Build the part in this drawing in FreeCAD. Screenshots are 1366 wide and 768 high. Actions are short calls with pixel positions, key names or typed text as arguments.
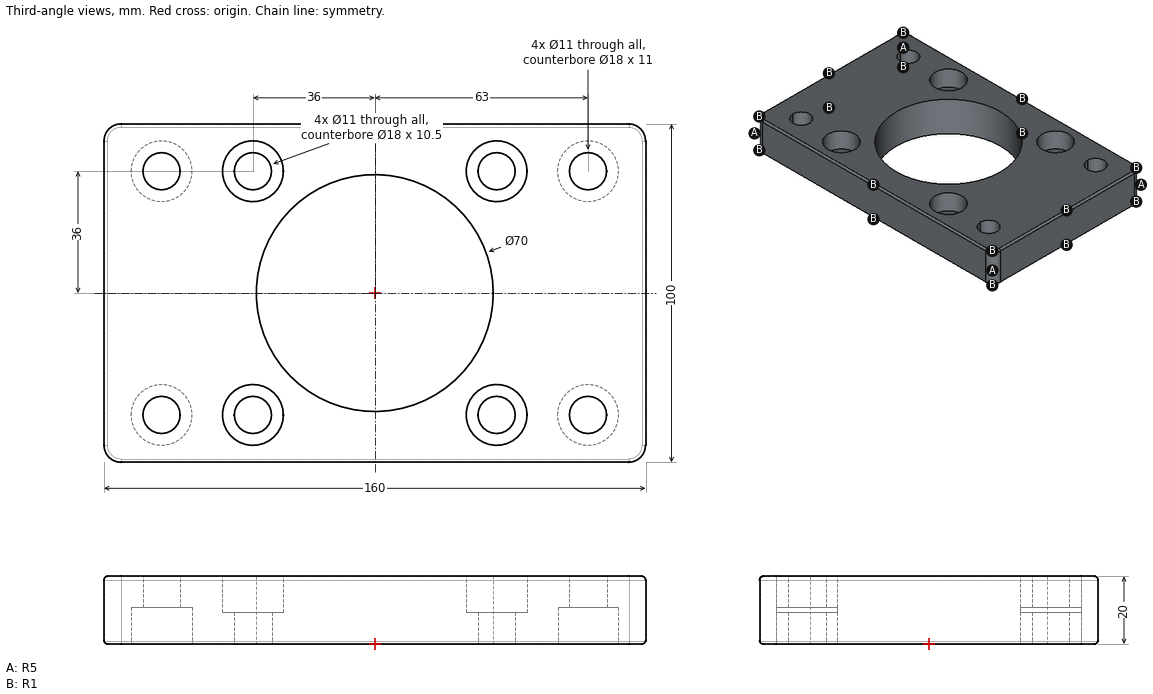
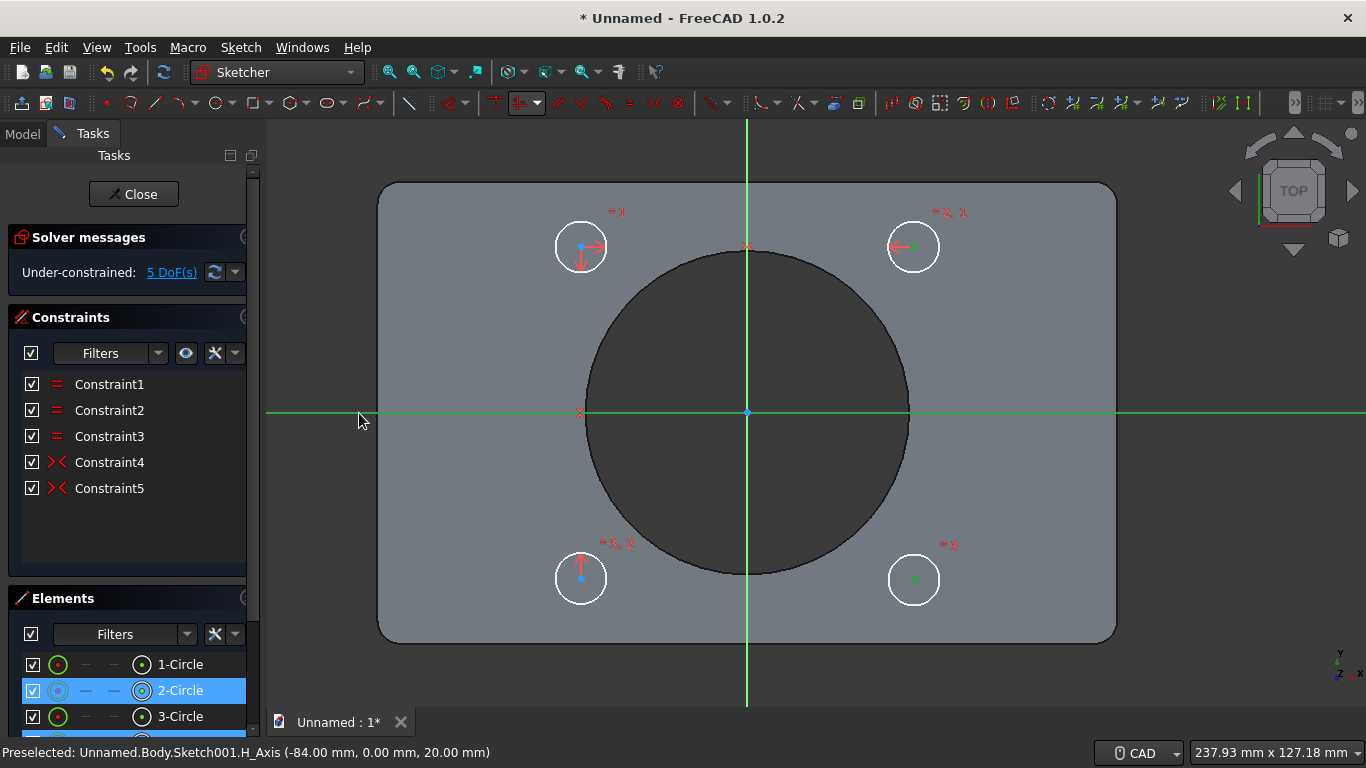
key(s)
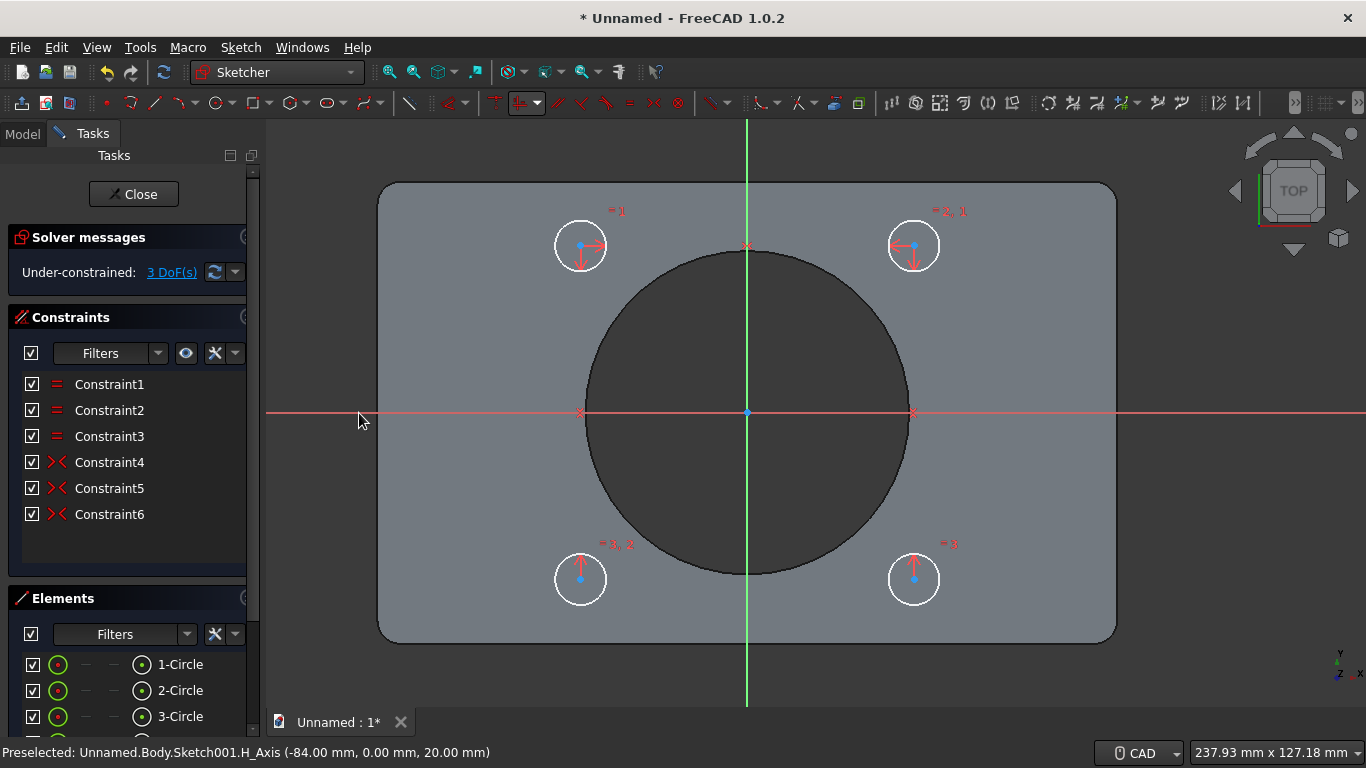
click(448, 104)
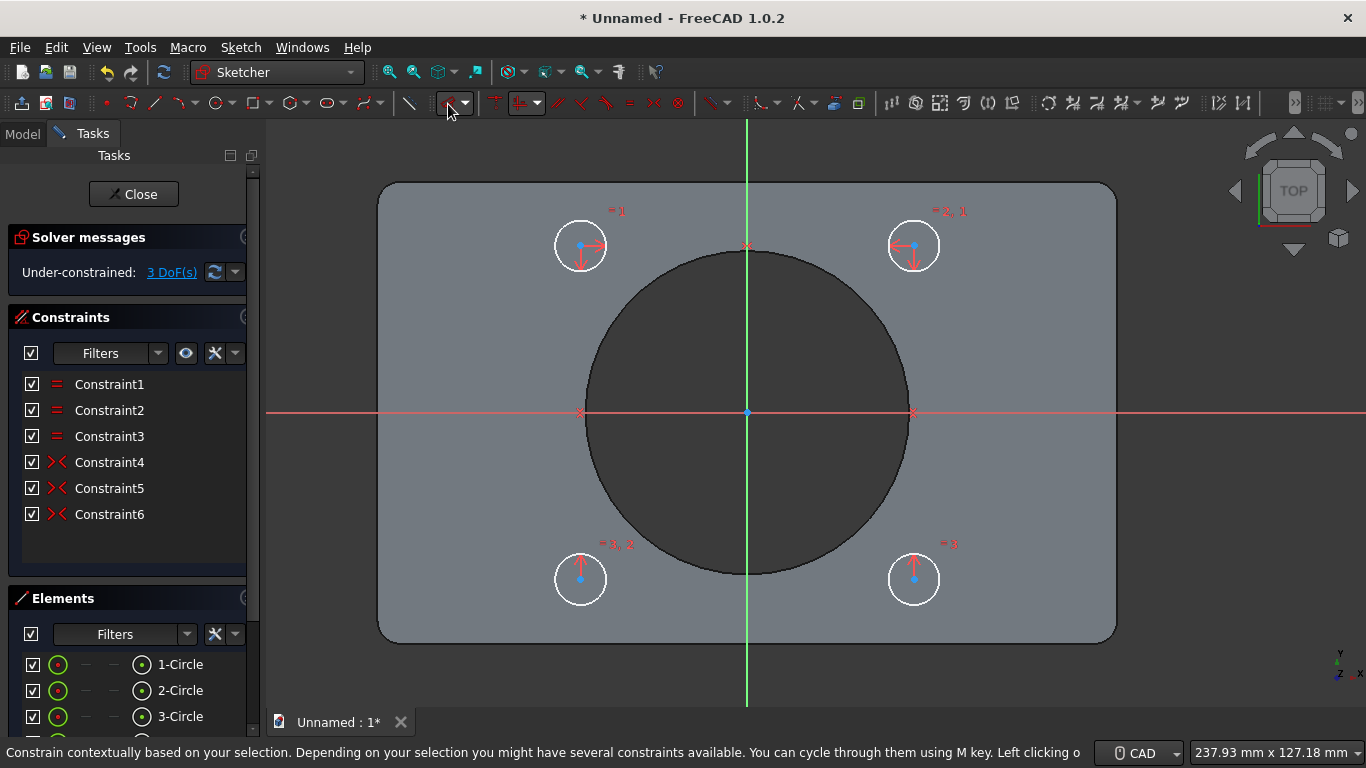
click(599, 228)
click(622, 206)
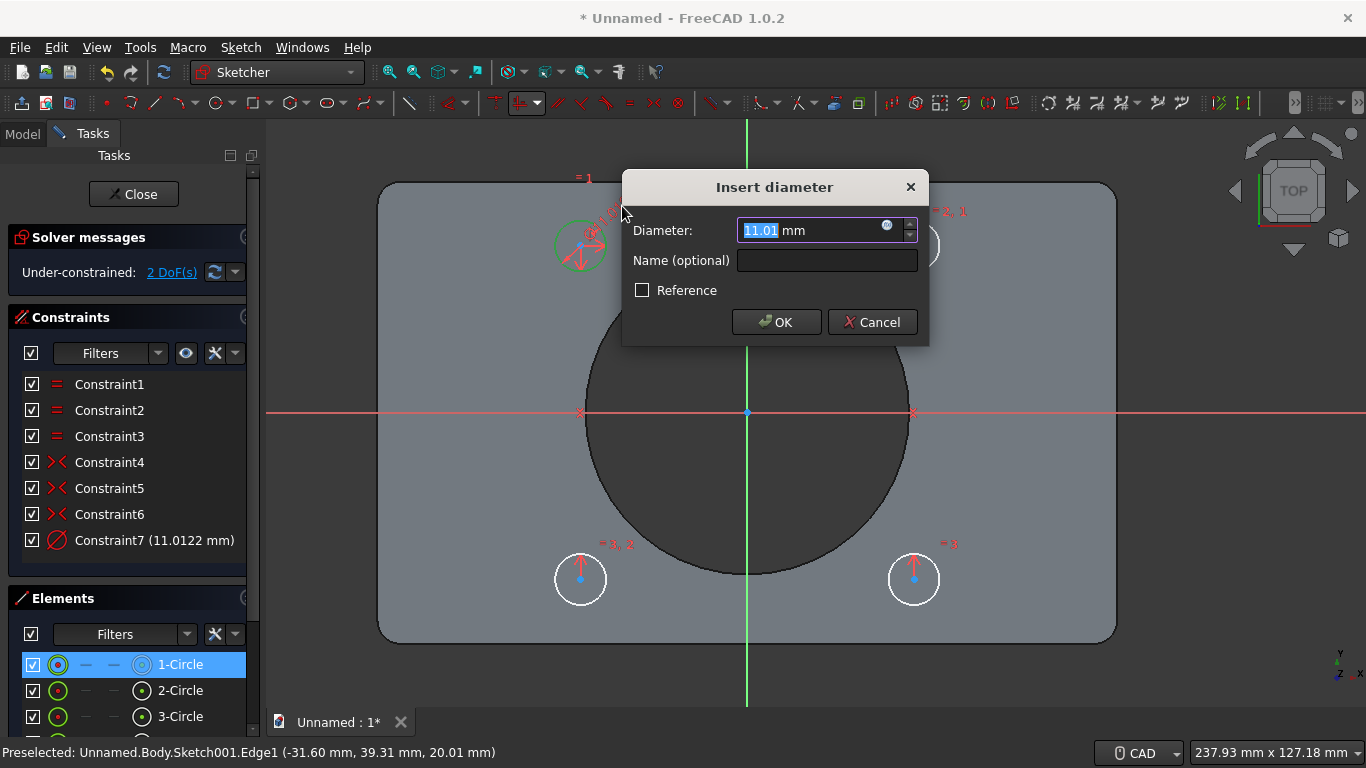
text(11)
key(Return)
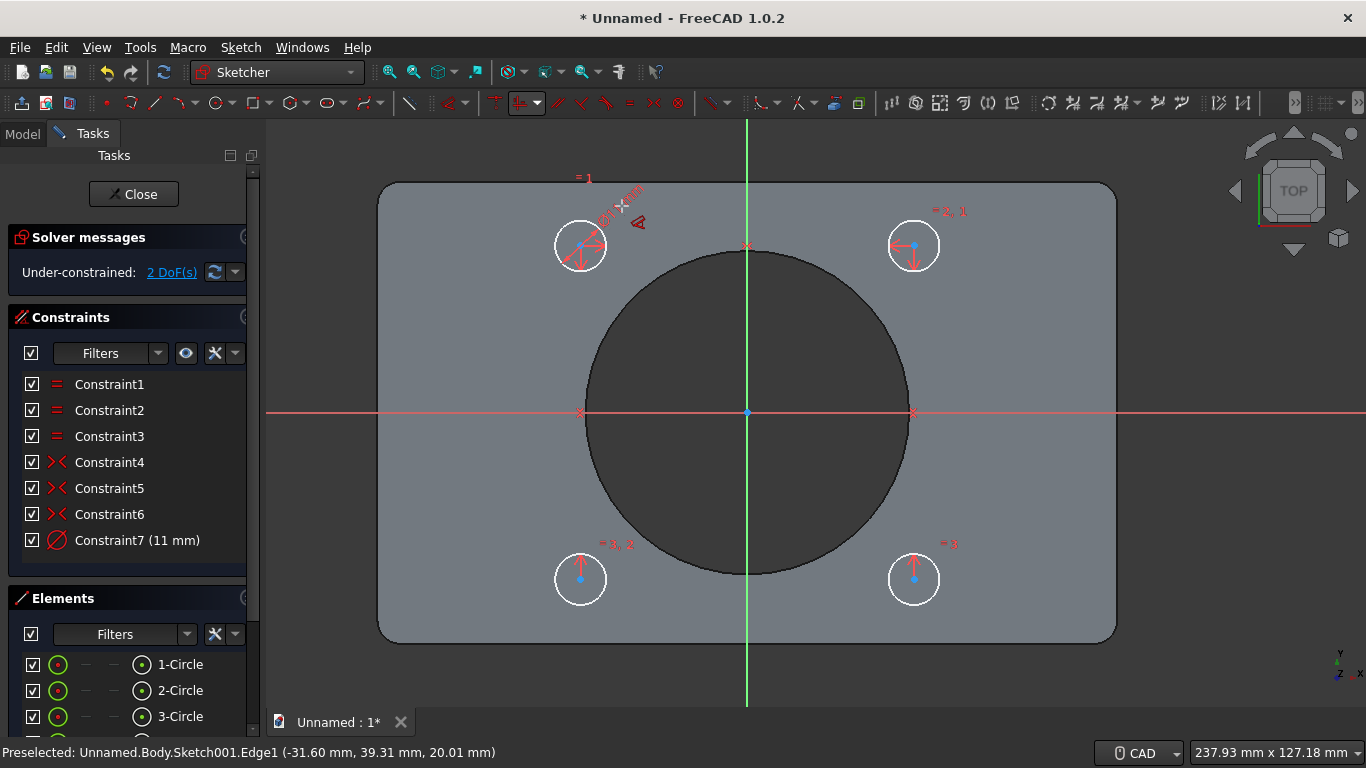
click(581, 246)
click(702, 212)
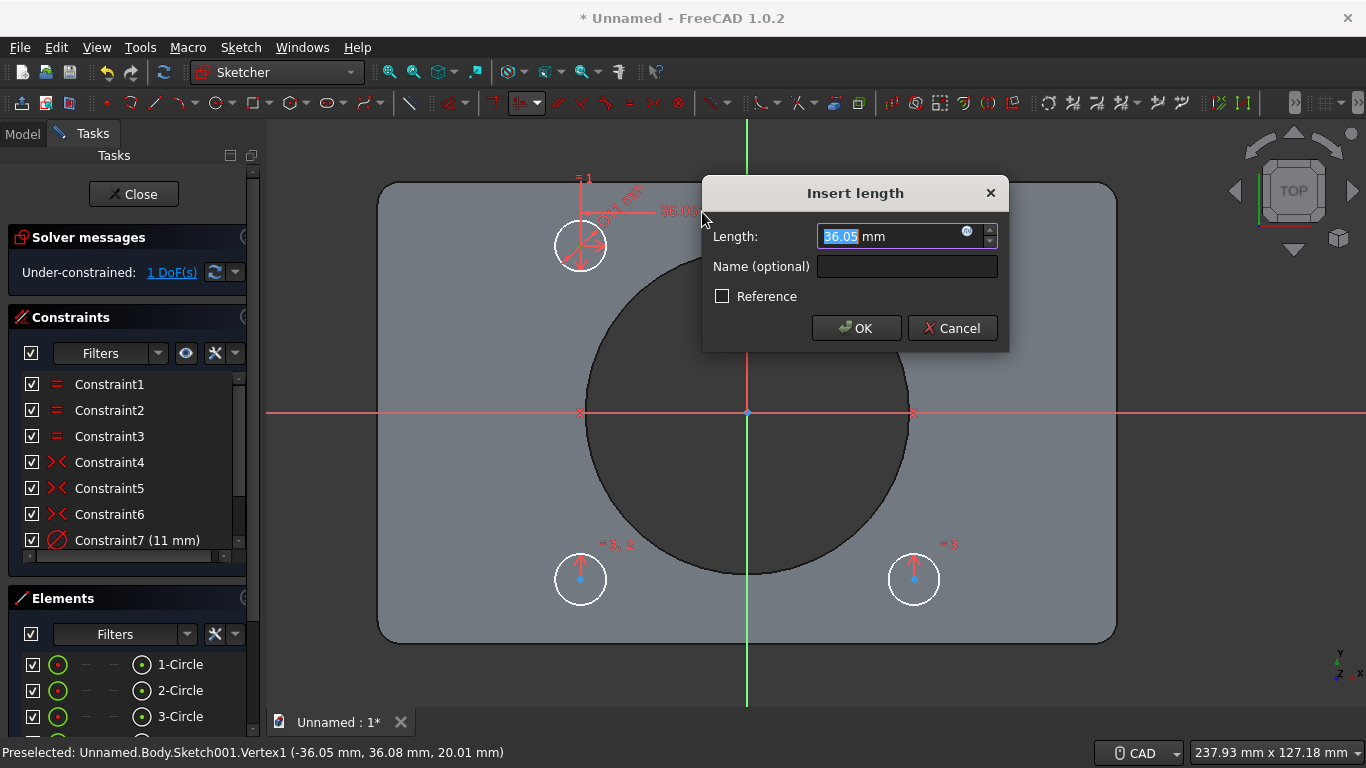
text(36)
key(Return)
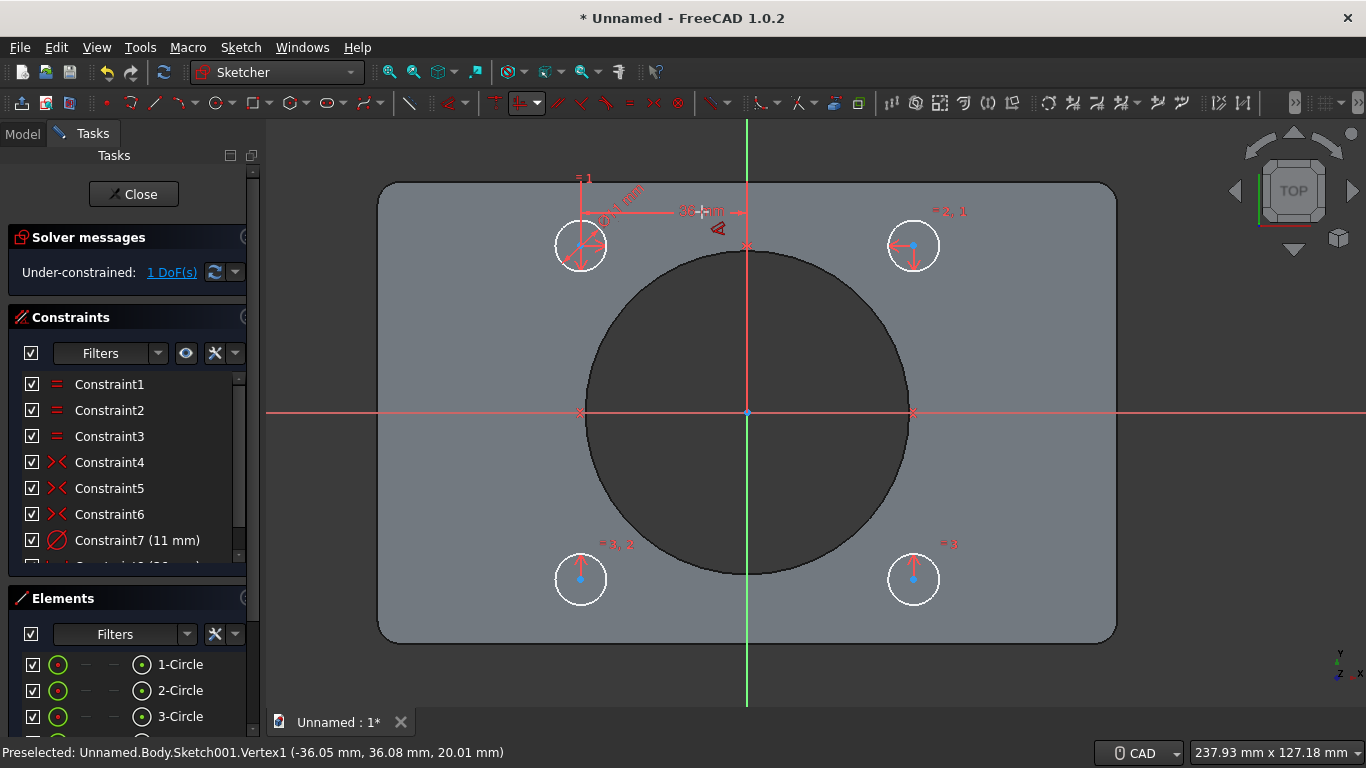
click(581, 246)
click(547, 329)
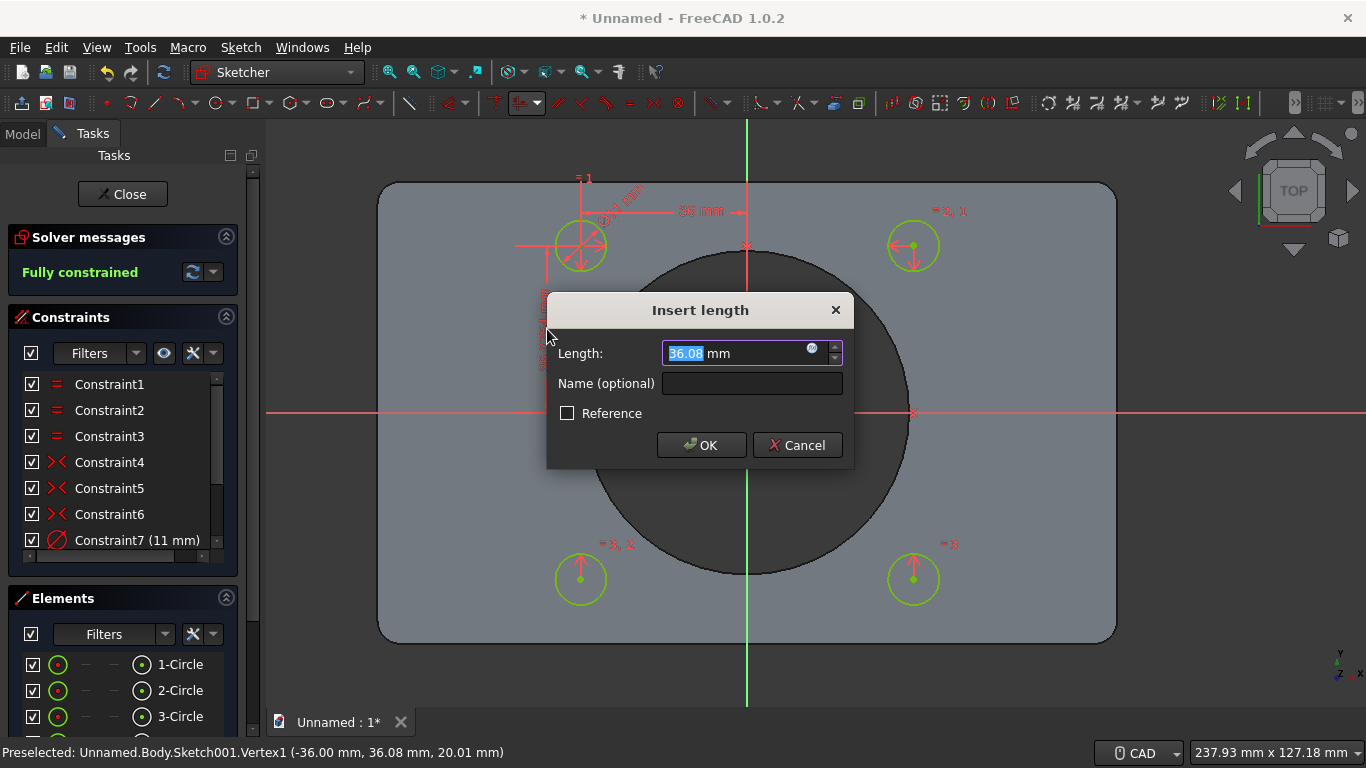
text(36)
key(Return)
key(Escape)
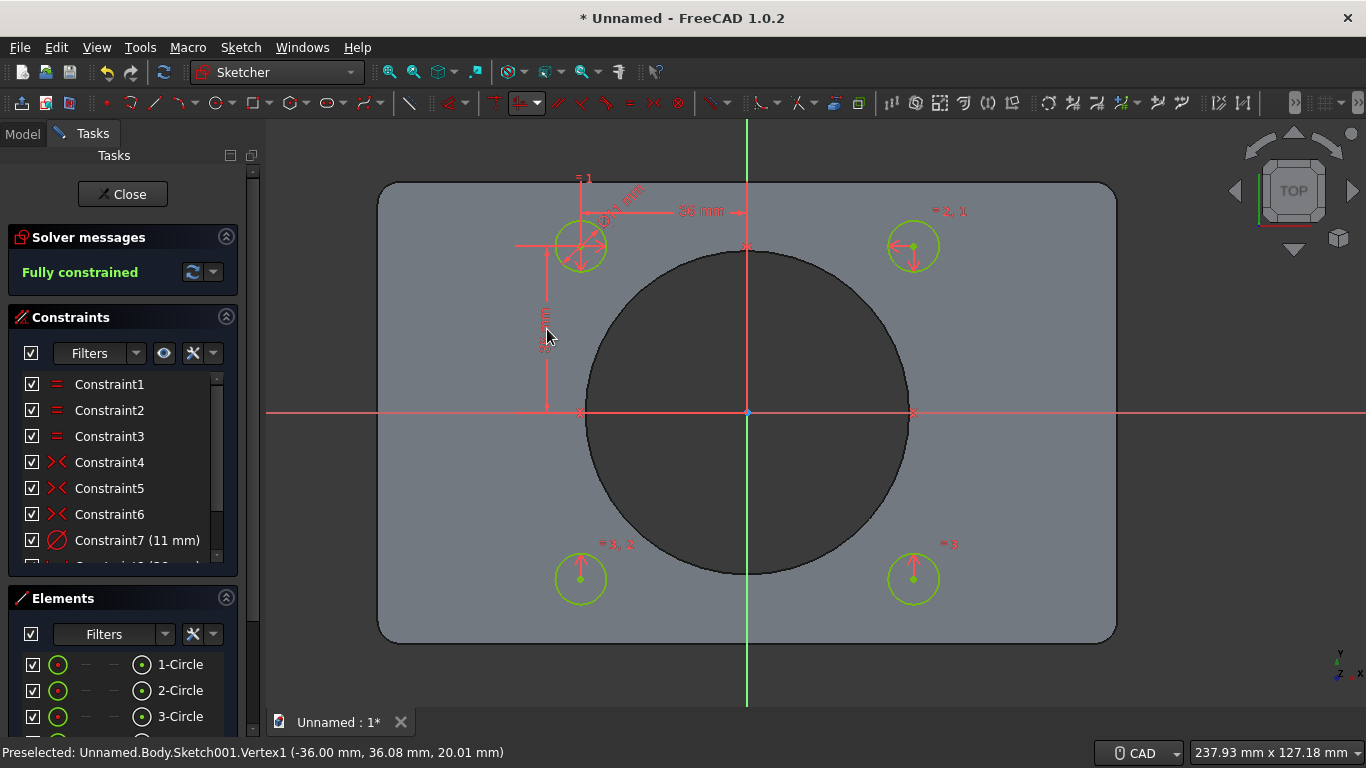
click(123, 194)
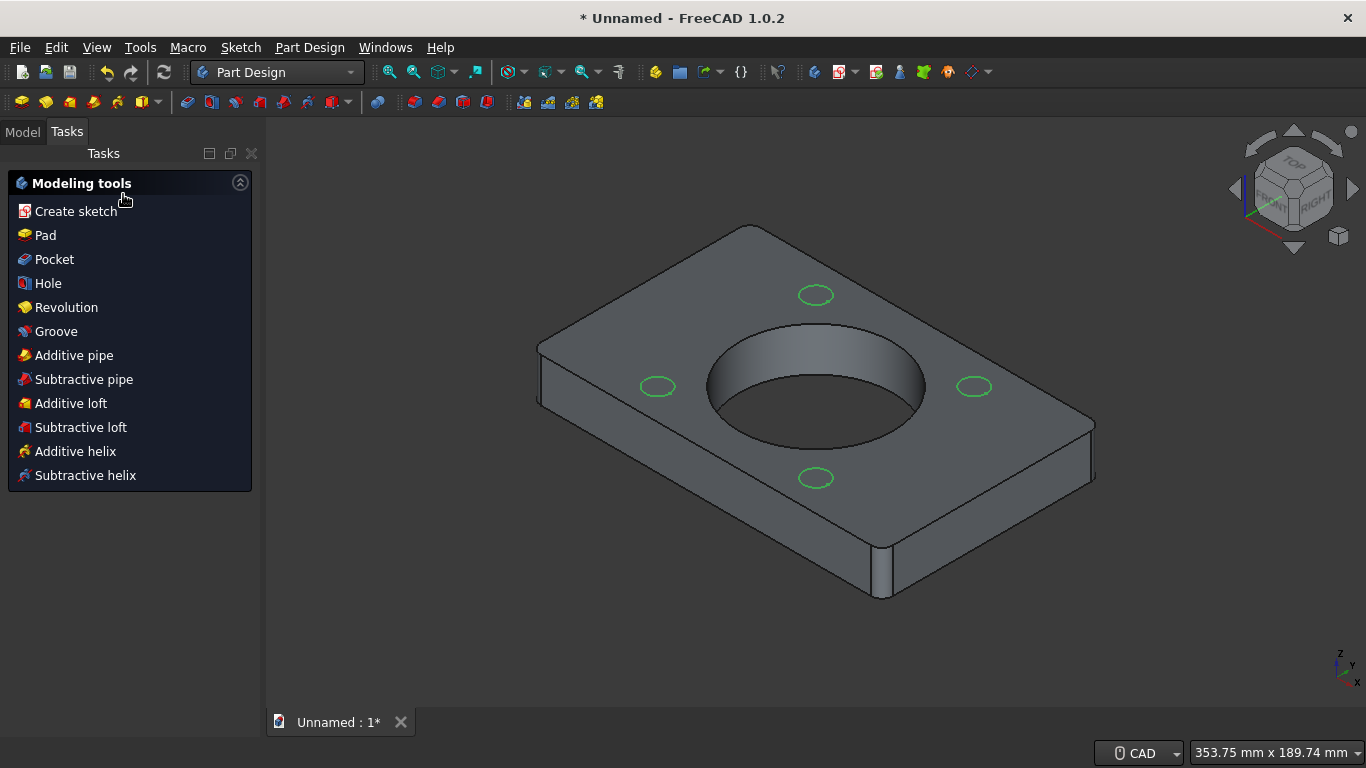
click(212, 102)